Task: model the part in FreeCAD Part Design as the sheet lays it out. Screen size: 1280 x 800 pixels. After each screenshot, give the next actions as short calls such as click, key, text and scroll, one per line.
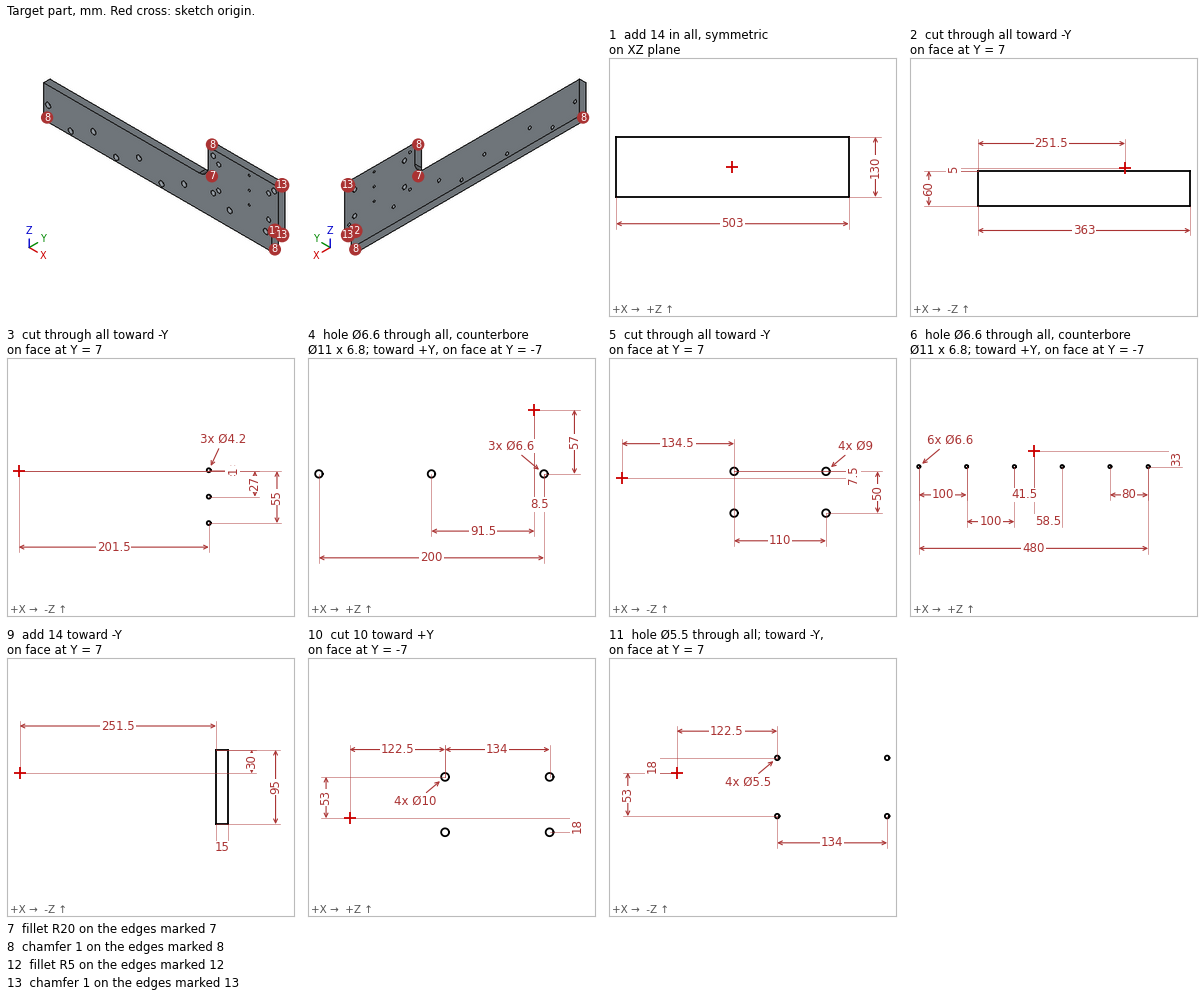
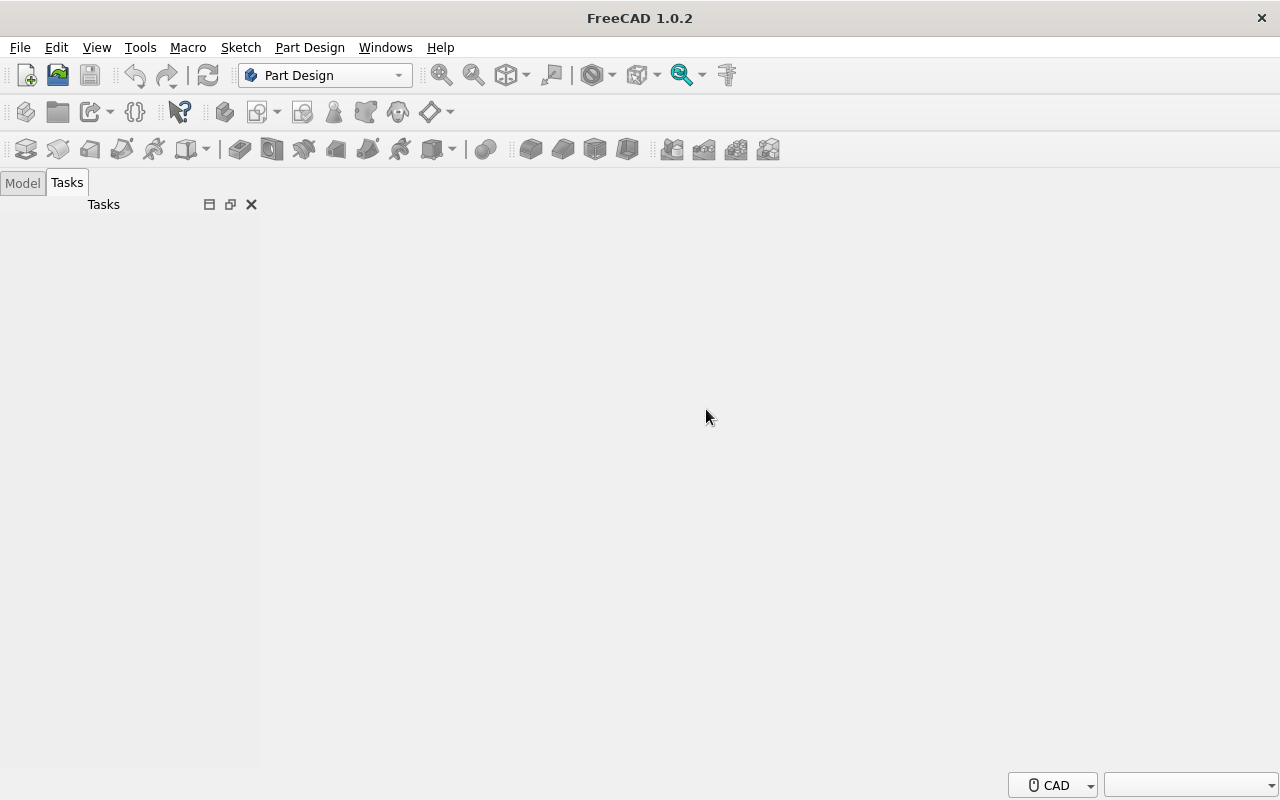
click(26, 76)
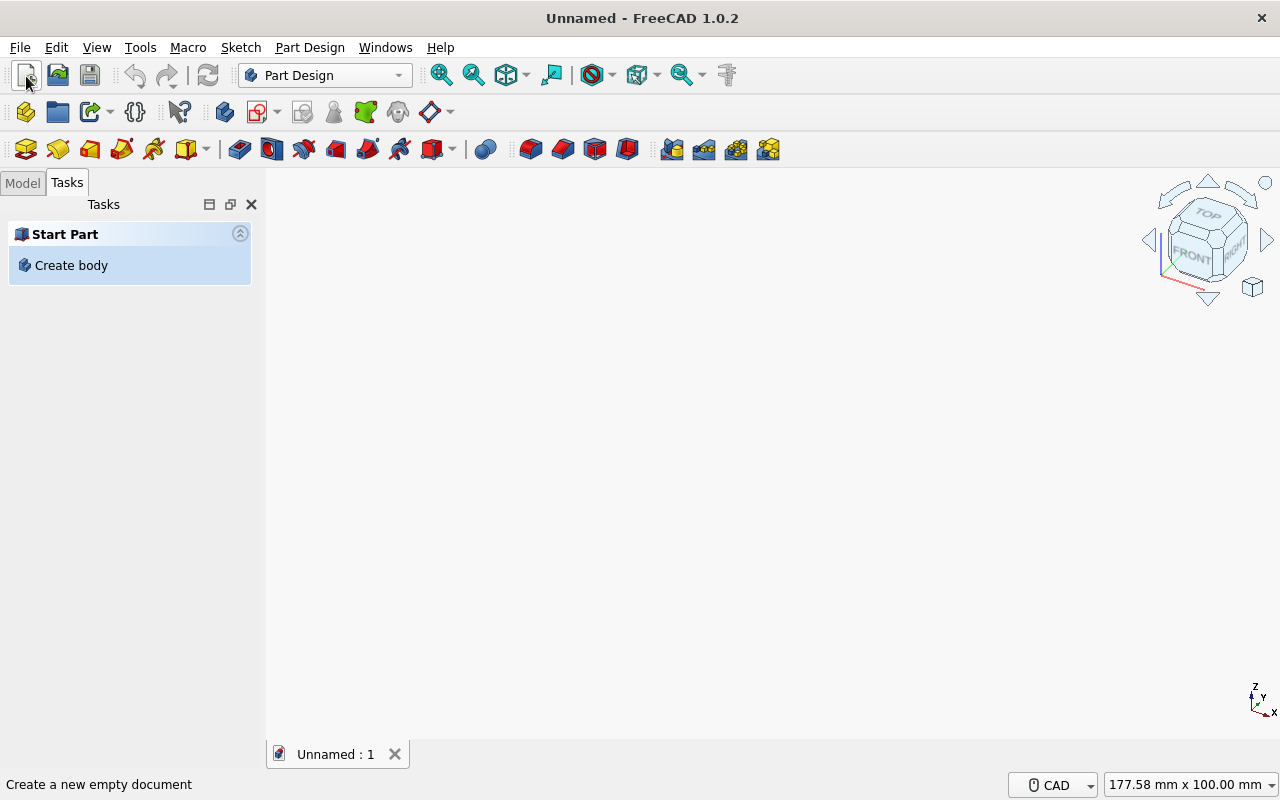
click(258, 112)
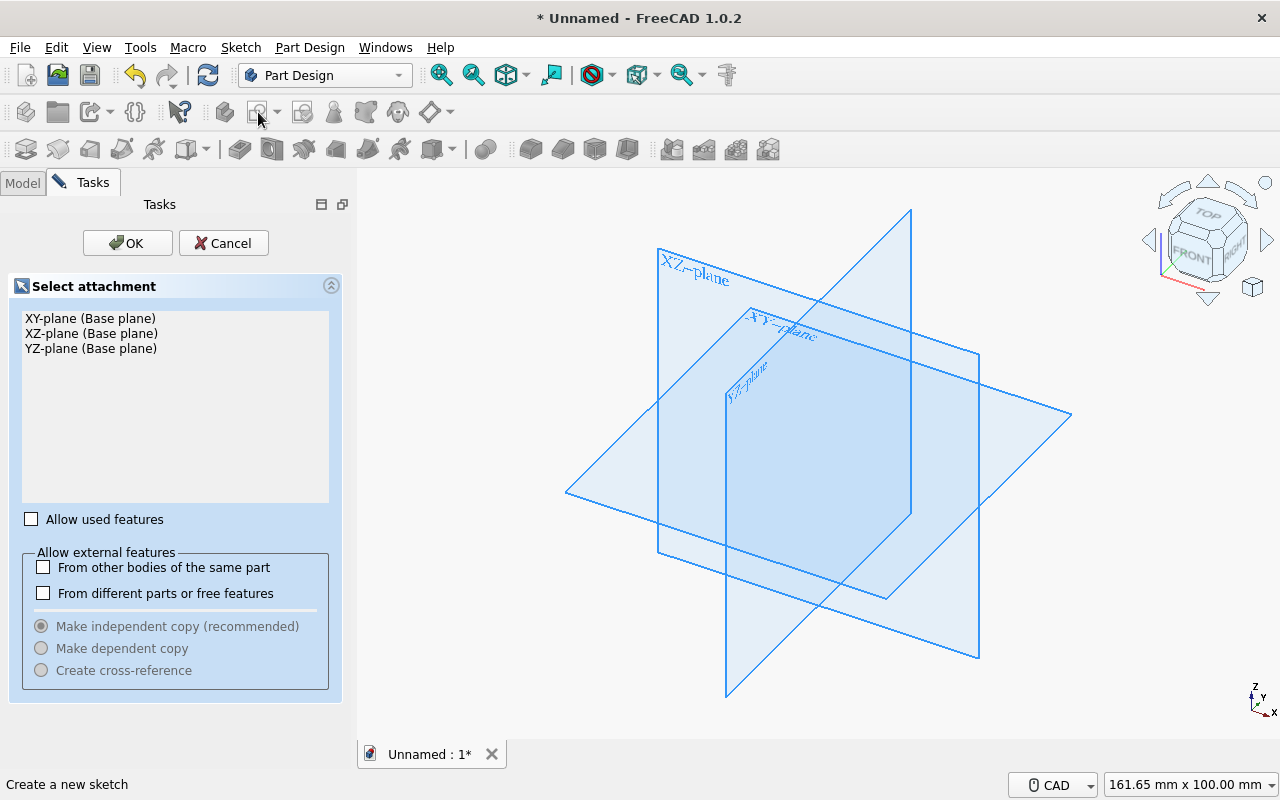
click(82, 334)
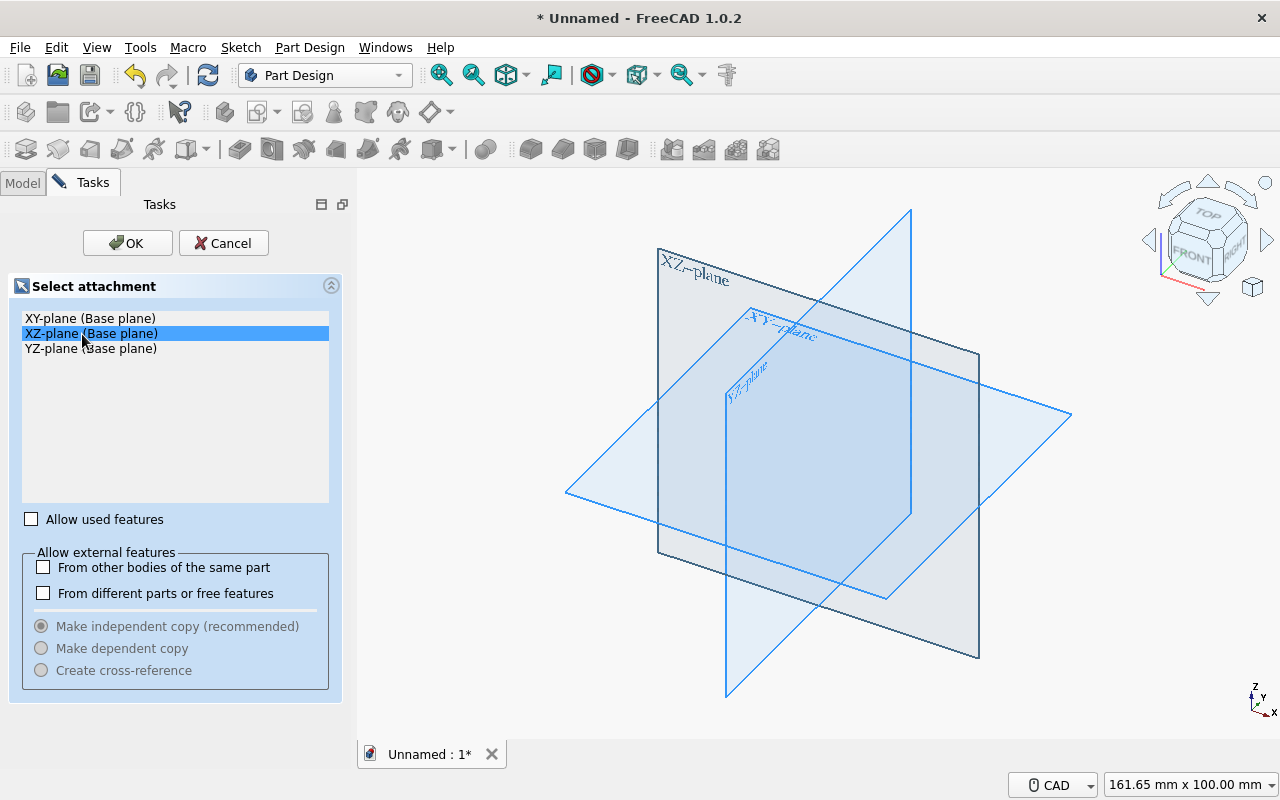
click(128, 243)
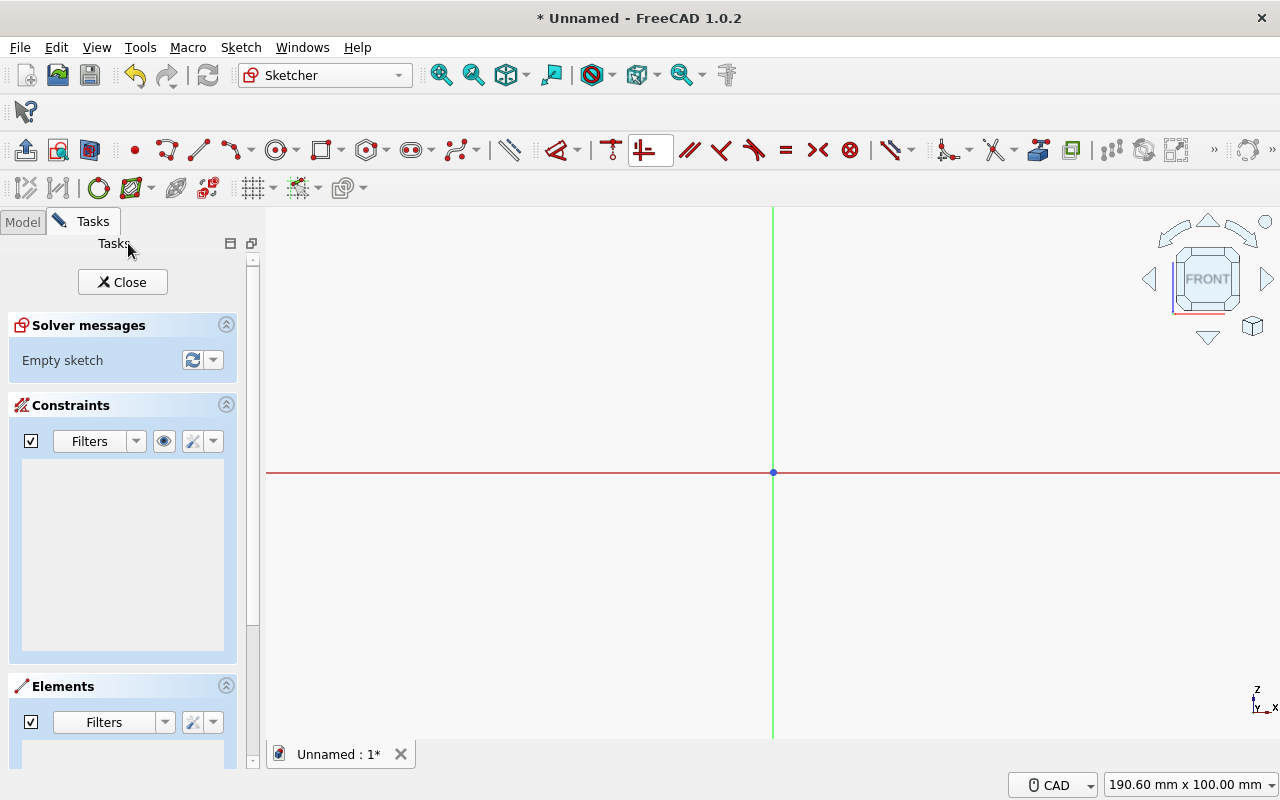
scroll(687, 473, down, 8)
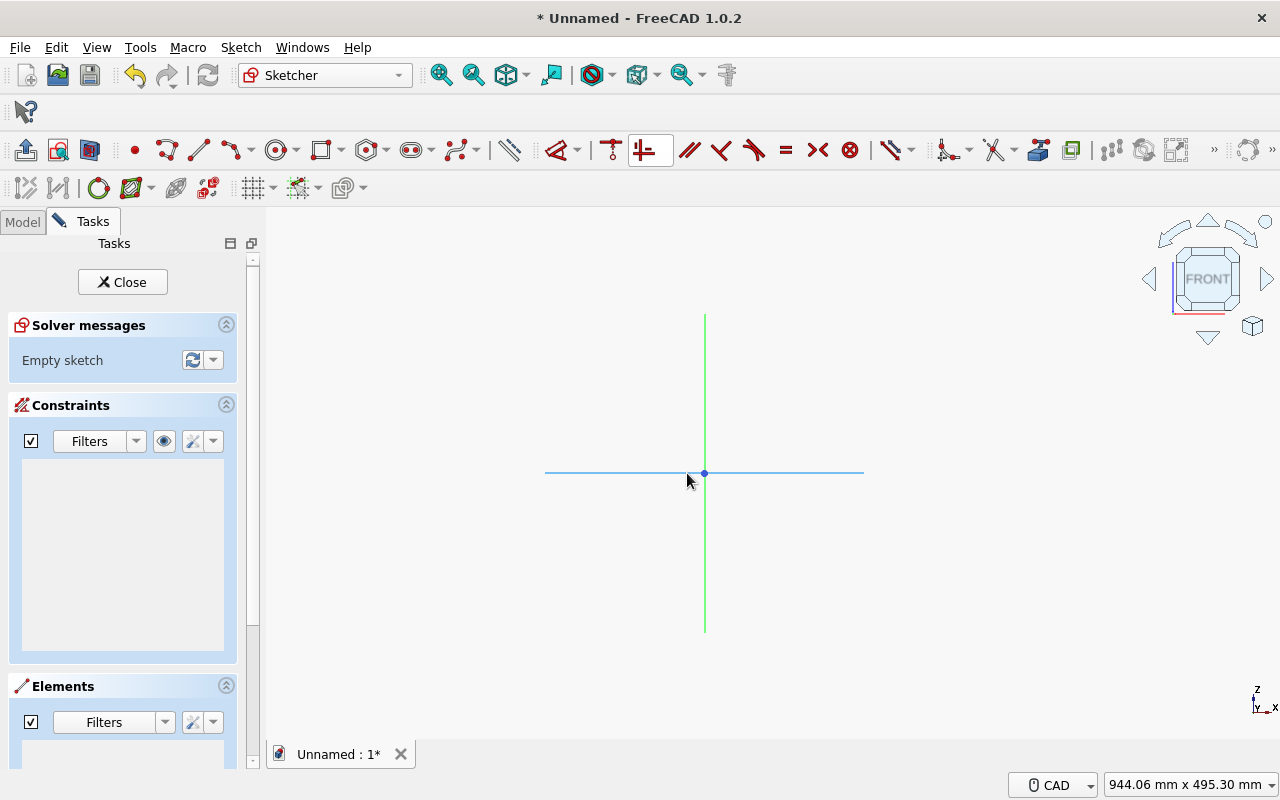
click(344, 150)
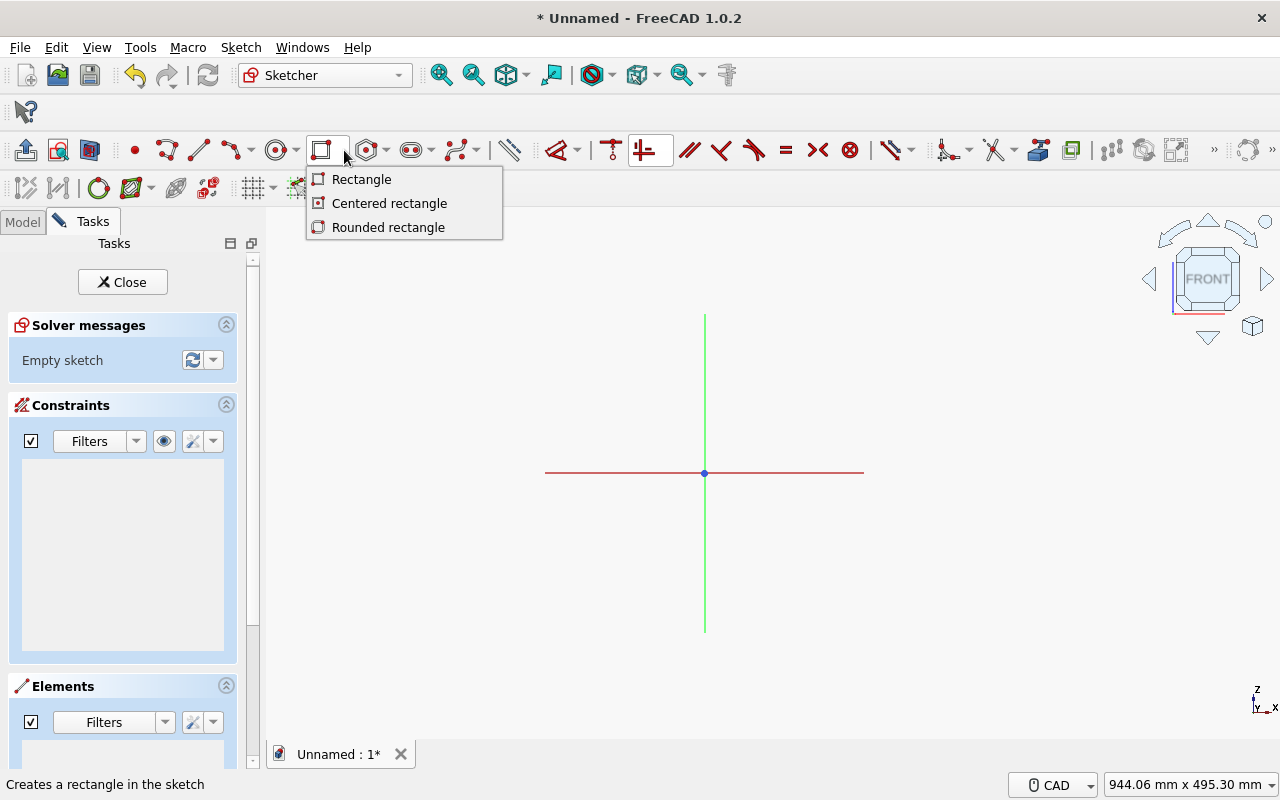
click(404, 203)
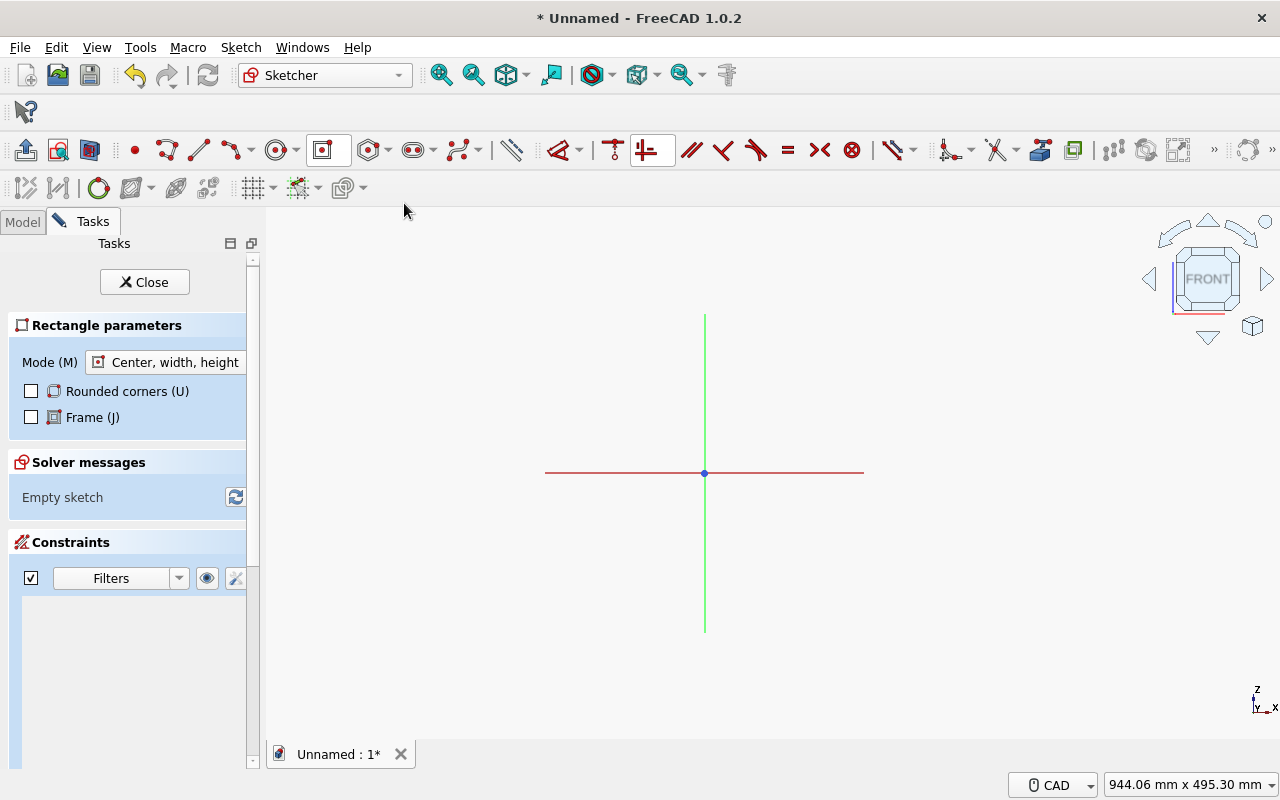
click(705, 473)
click(975, 404)
key(Escape)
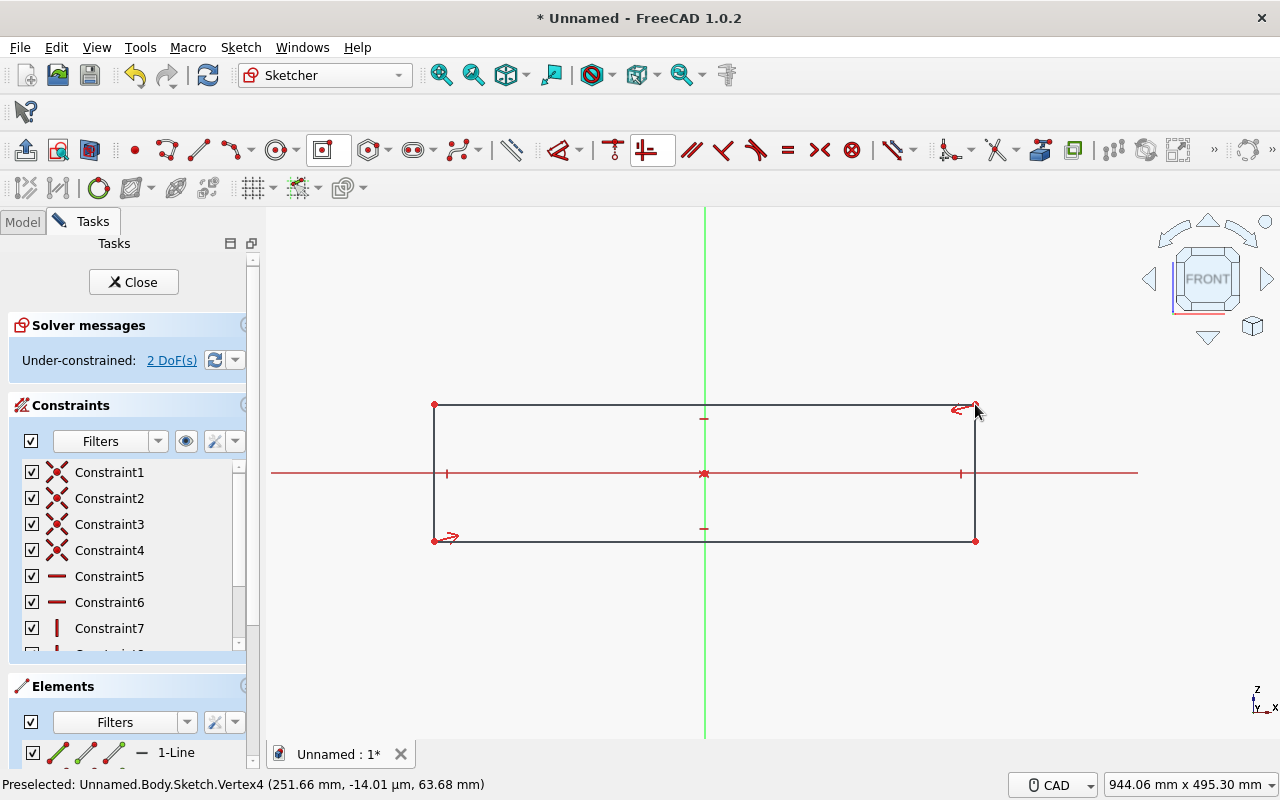
click(597, 542)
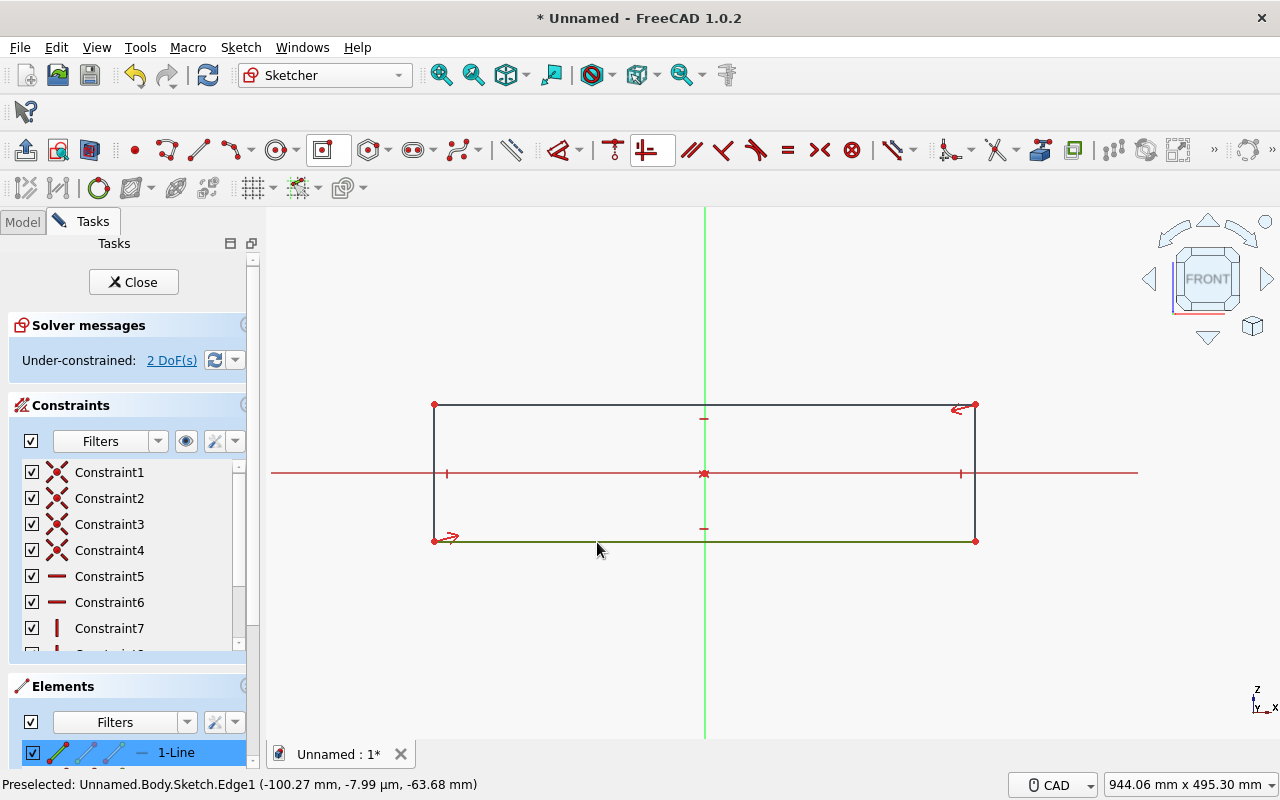
key(l)